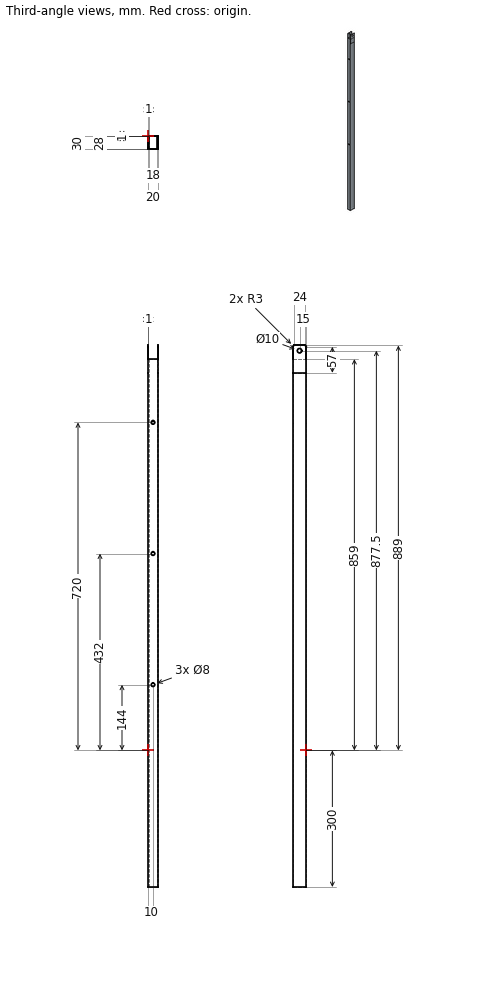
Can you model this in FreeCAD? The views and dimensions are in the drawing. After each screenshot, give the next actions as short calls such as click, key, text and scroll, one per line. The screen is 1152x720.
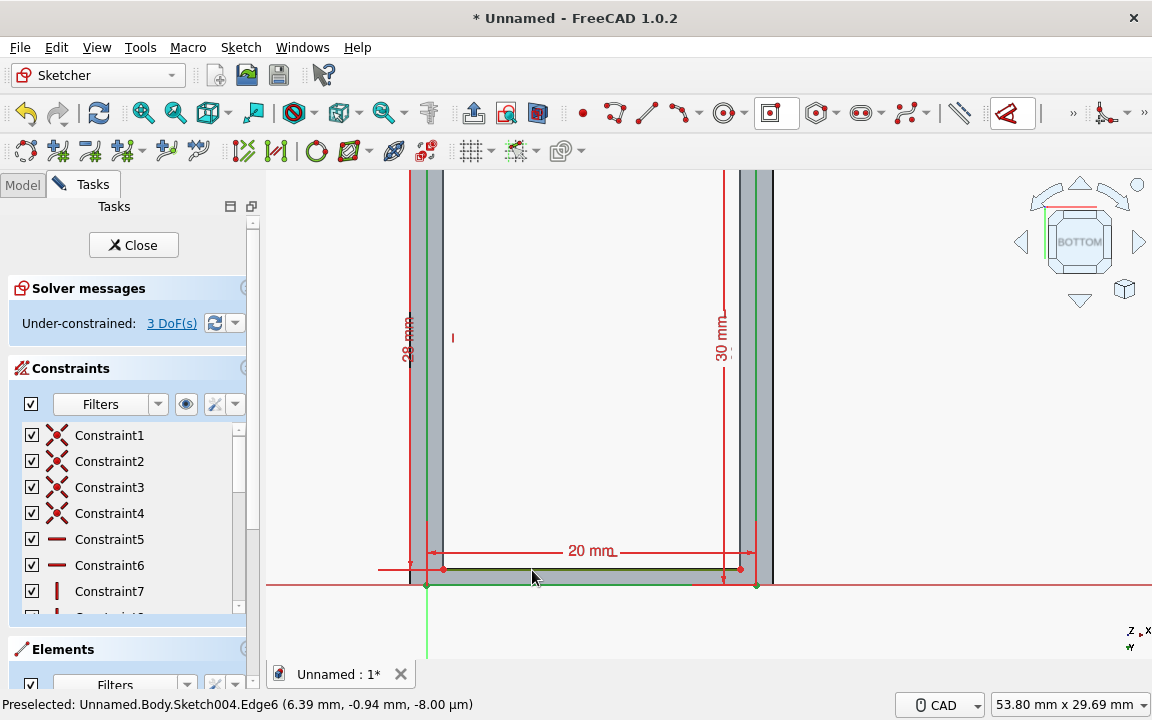
key(l)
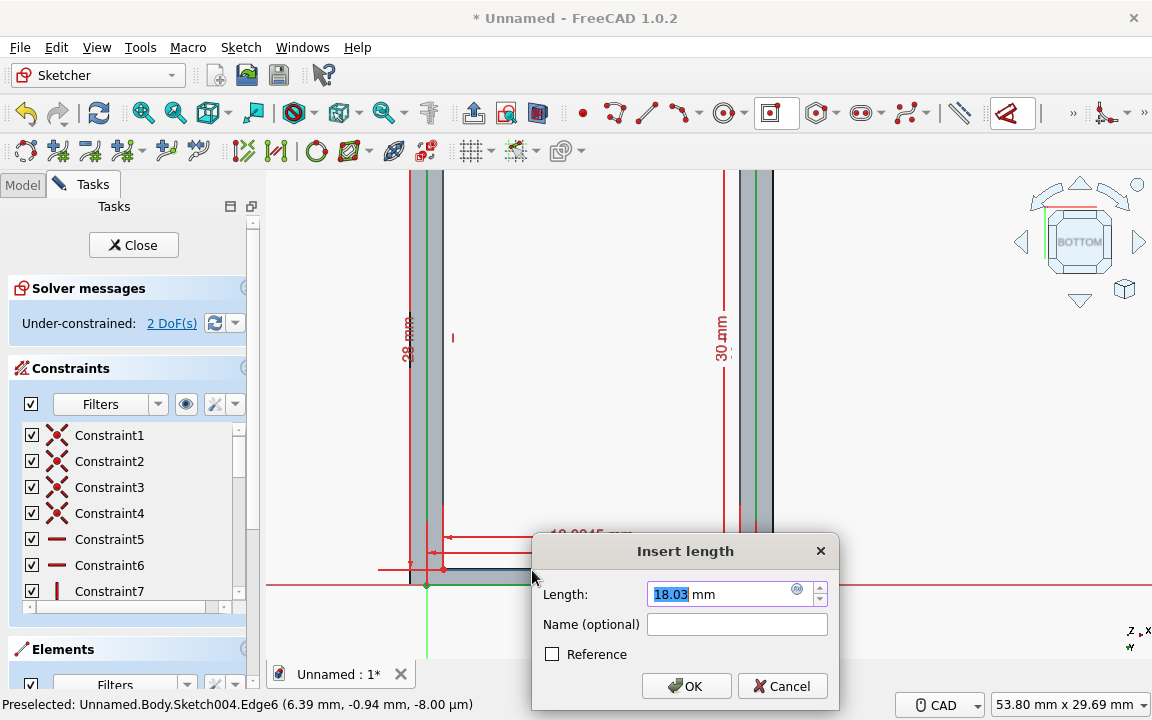
text(18)
key(Return)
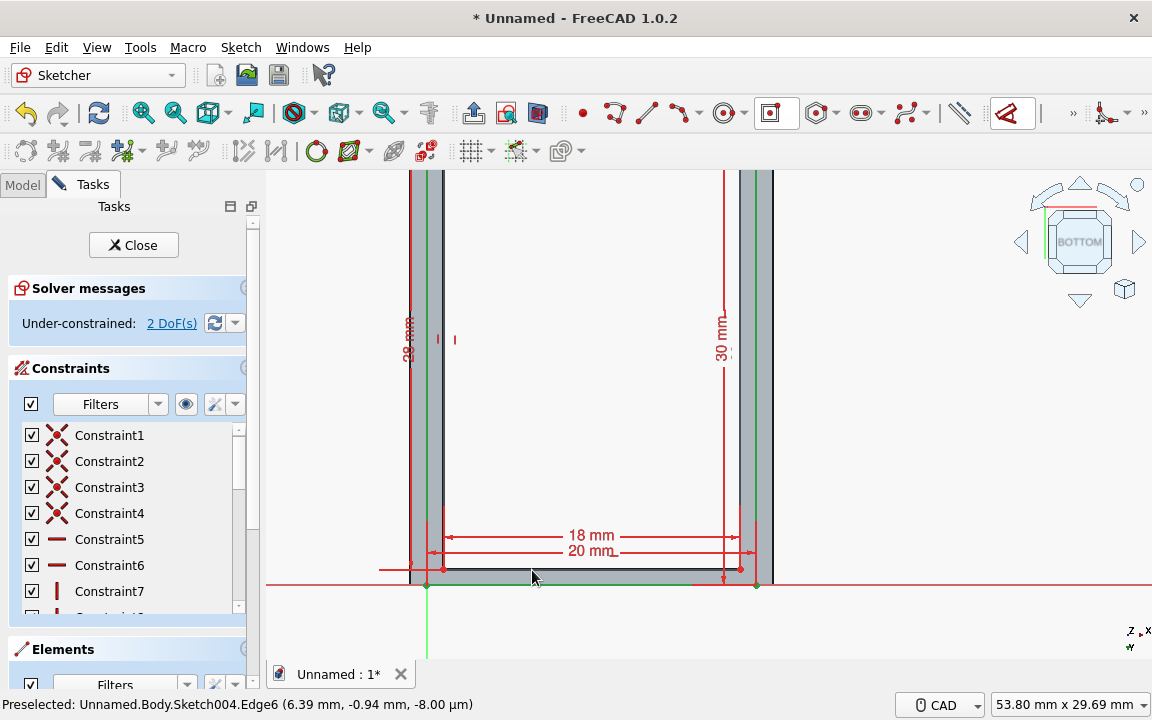
scroll(740, 569, down, 2)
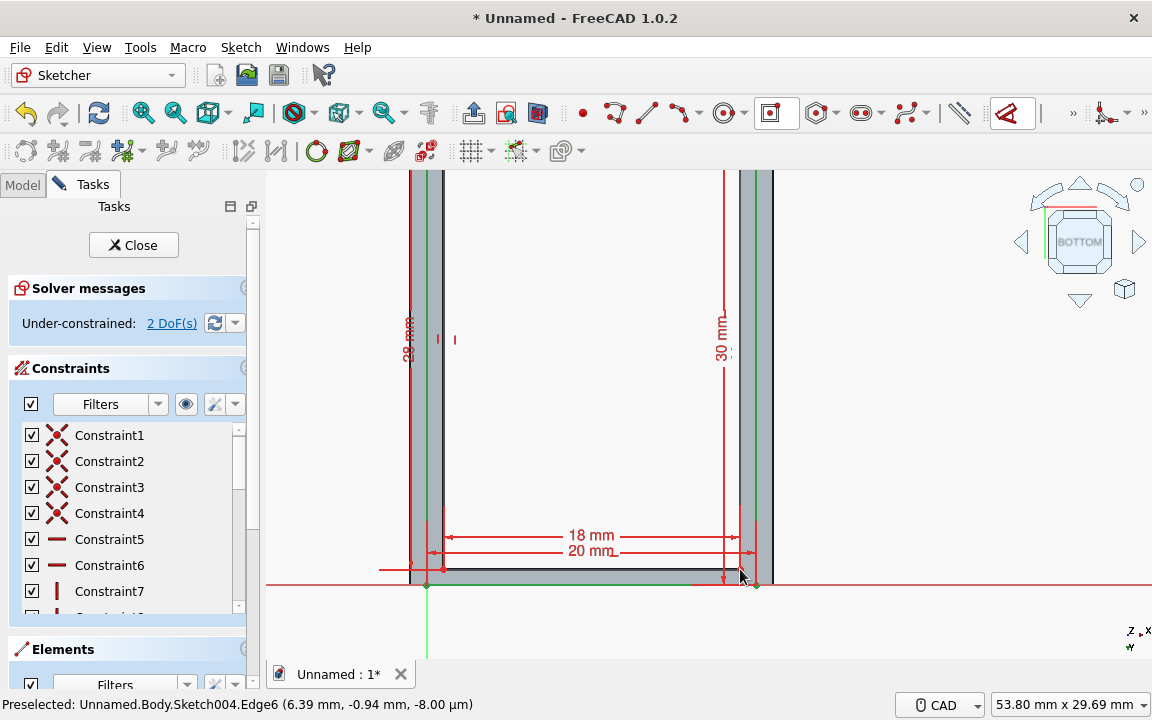
scroll(541, 261, up, 7)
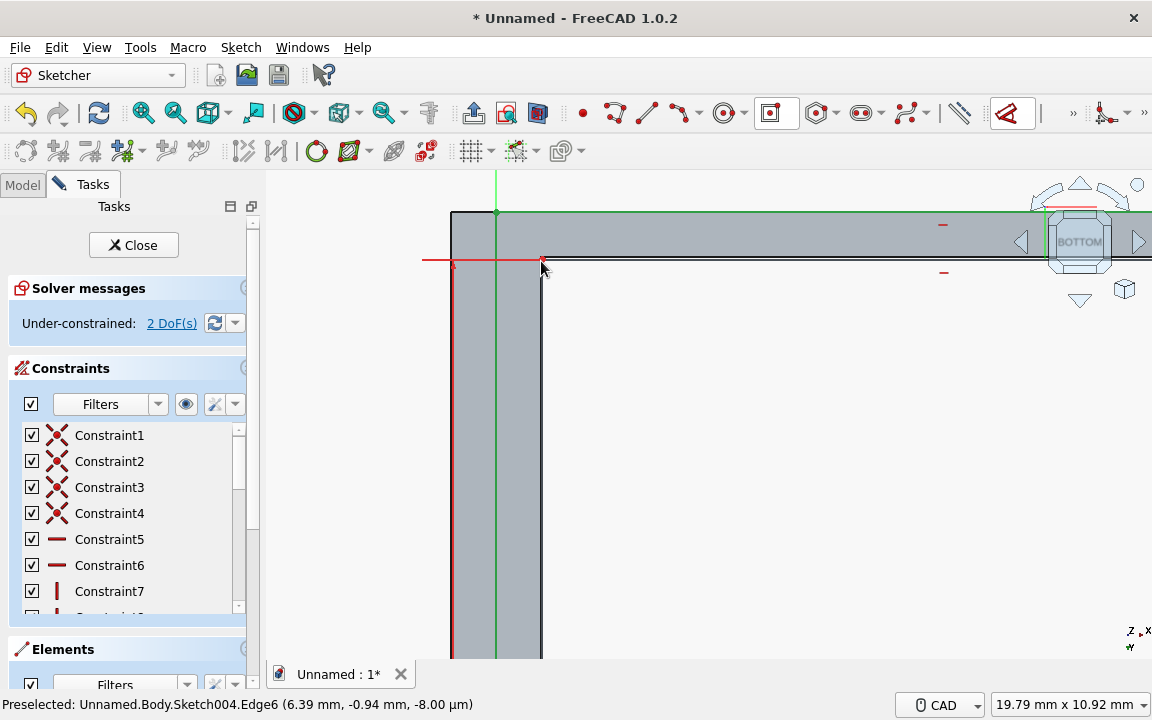
click(542, 260)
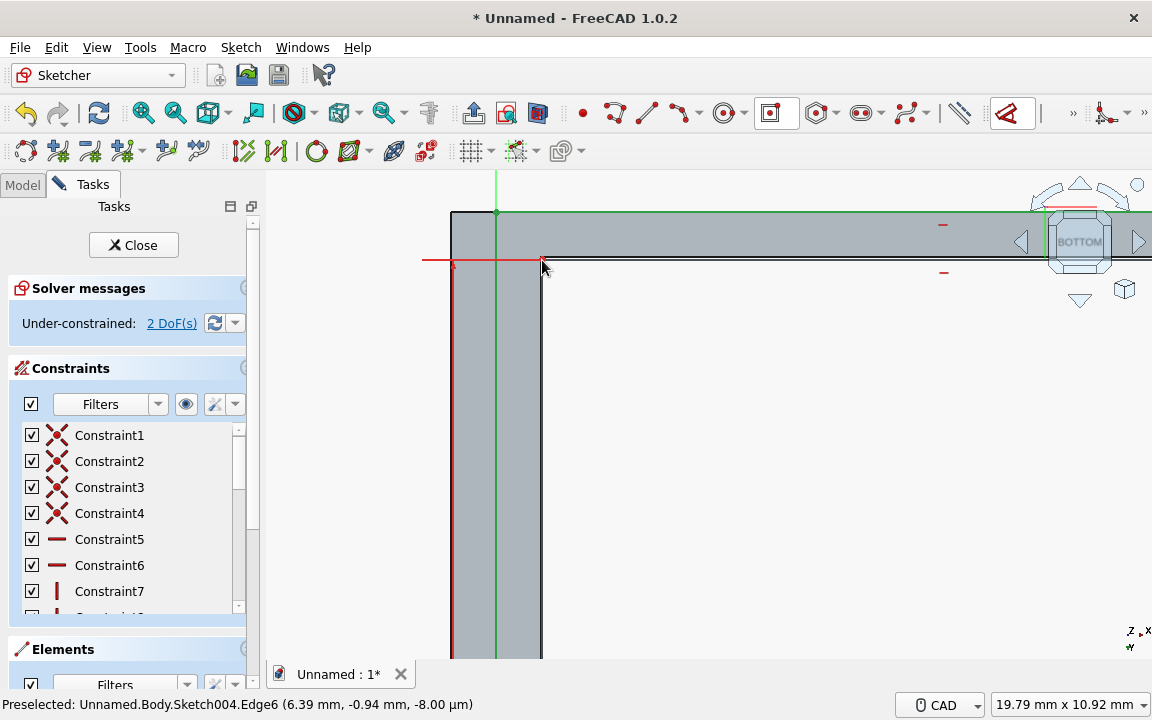
key(l)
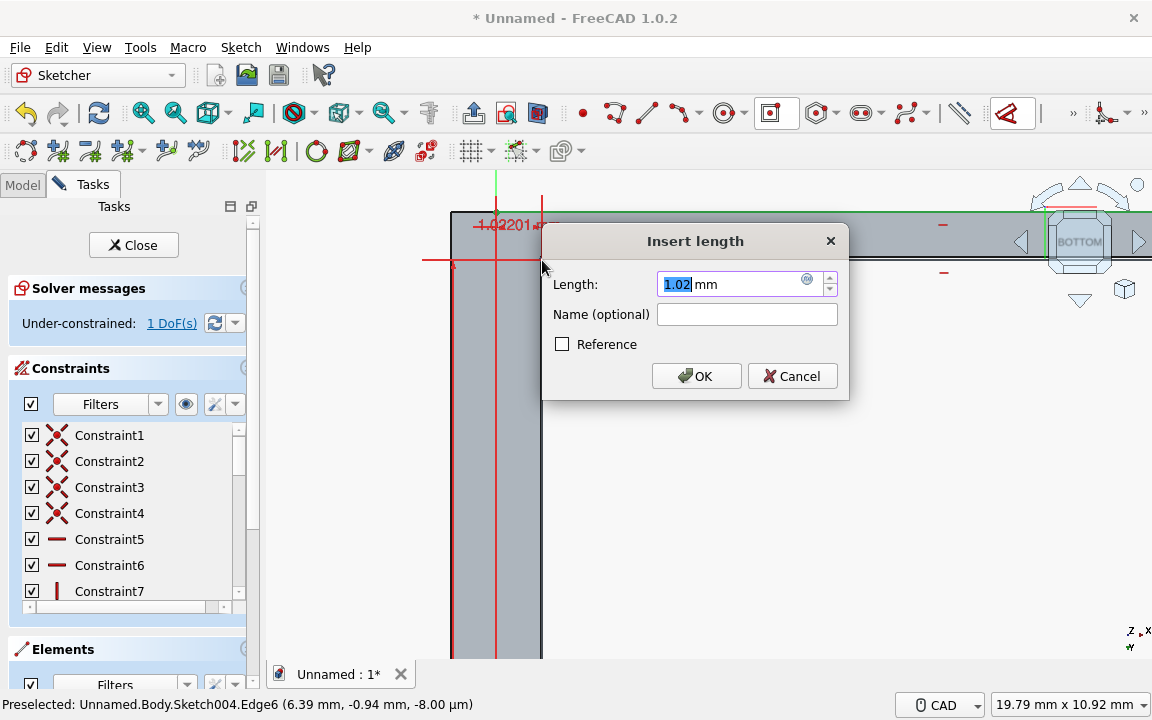
text(1)
key(Return)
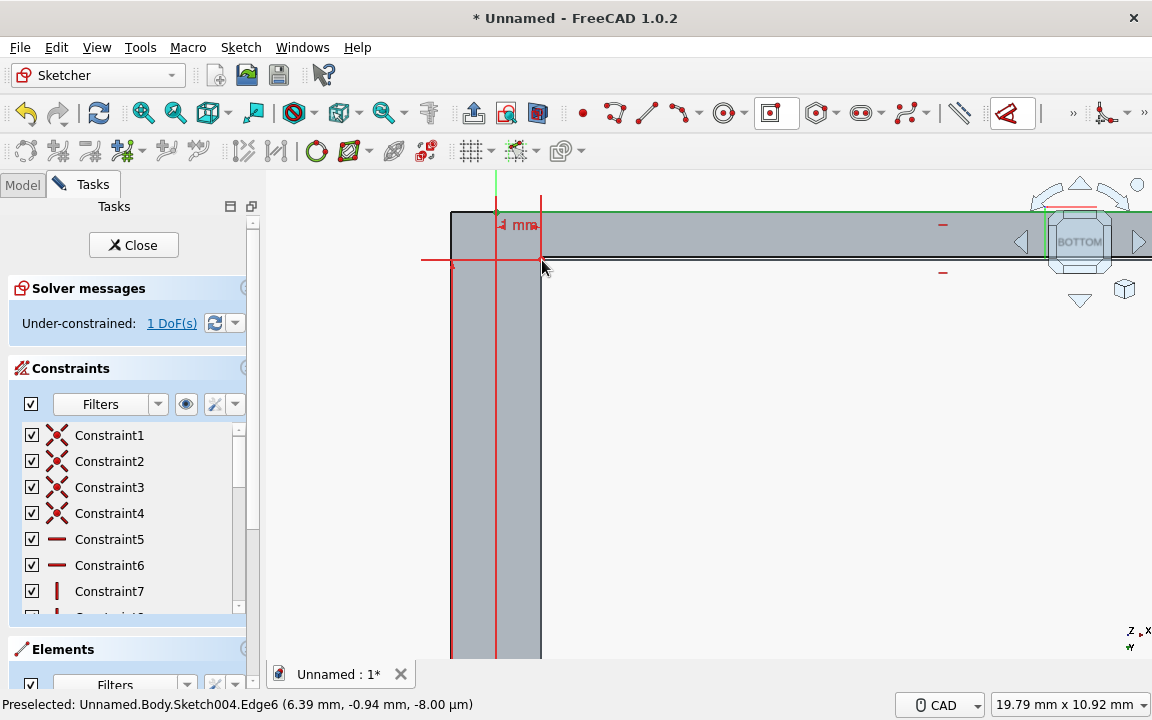
scroll(541, 261, down, 7)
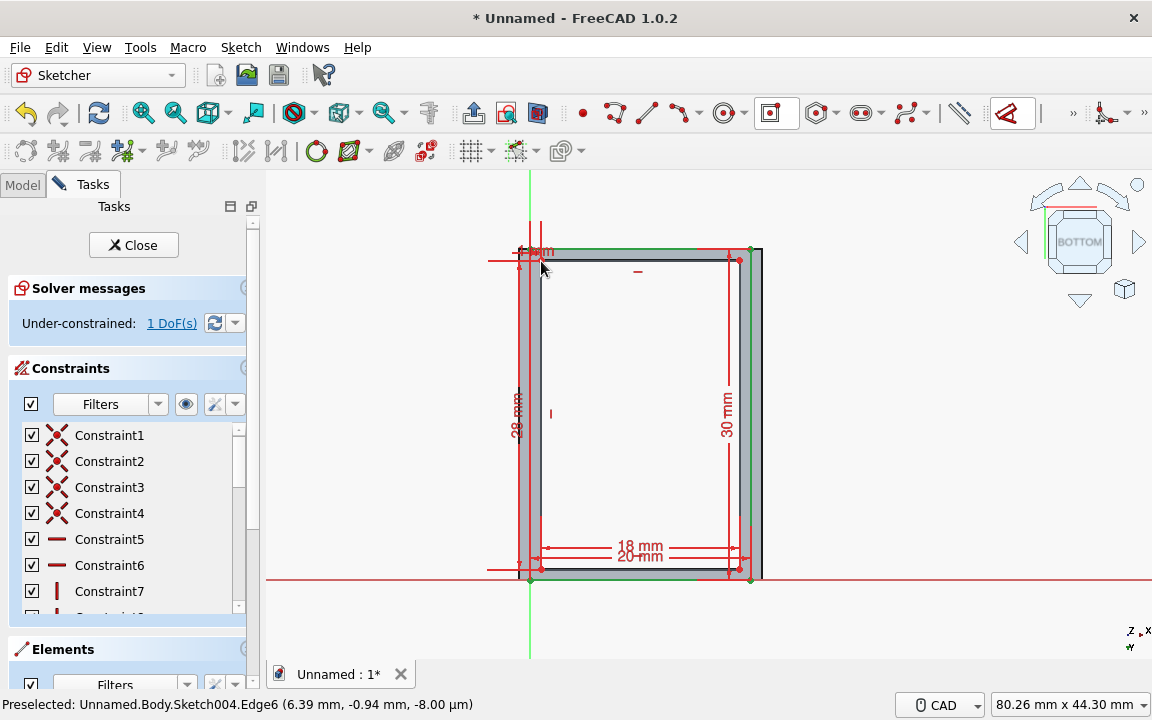
scroll(541, 570, up, 7)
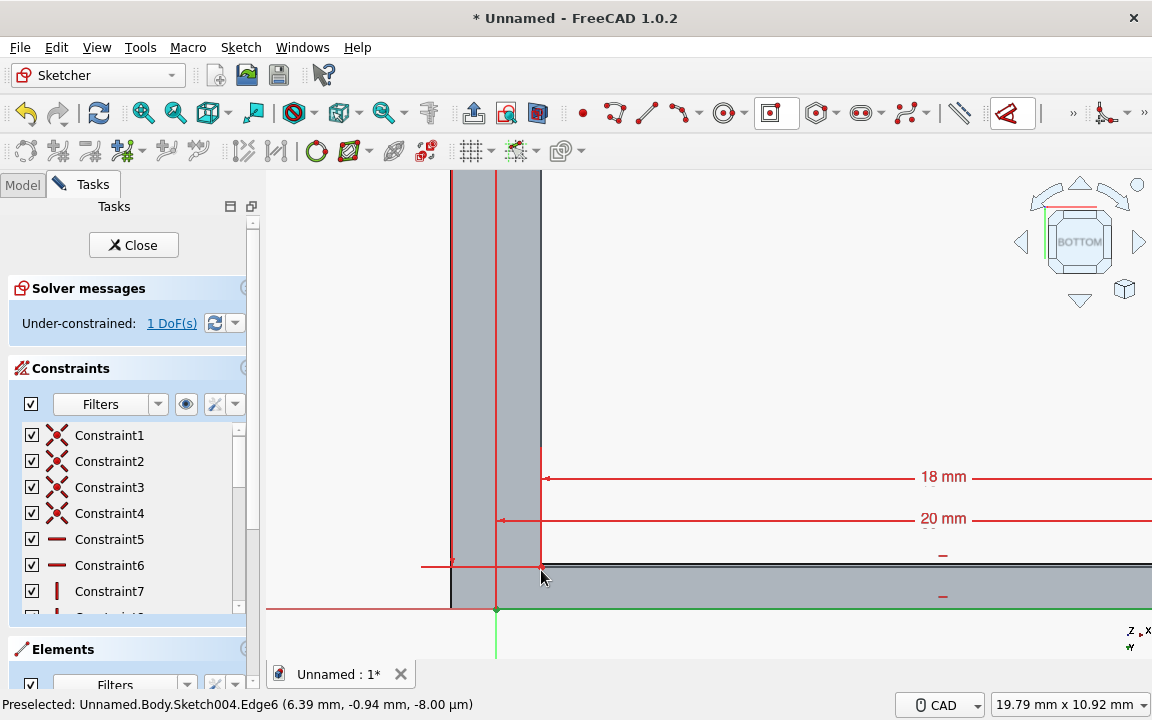
click(541, 567)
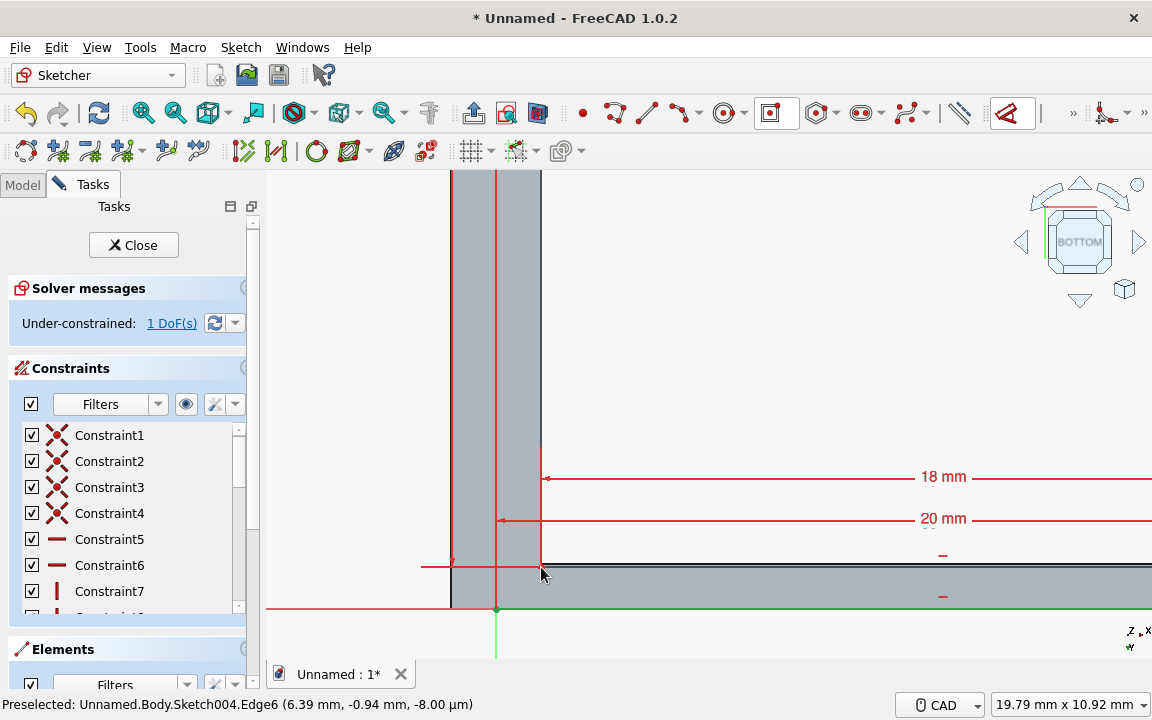
click(1030, 114)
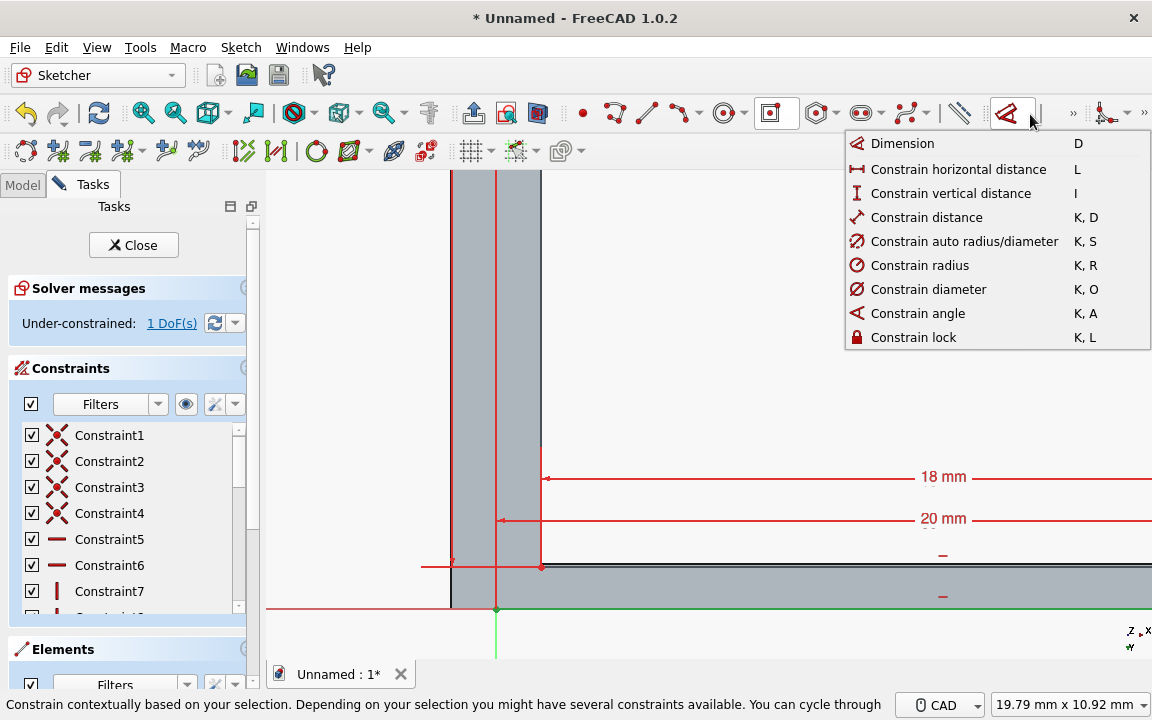
click(998, 193)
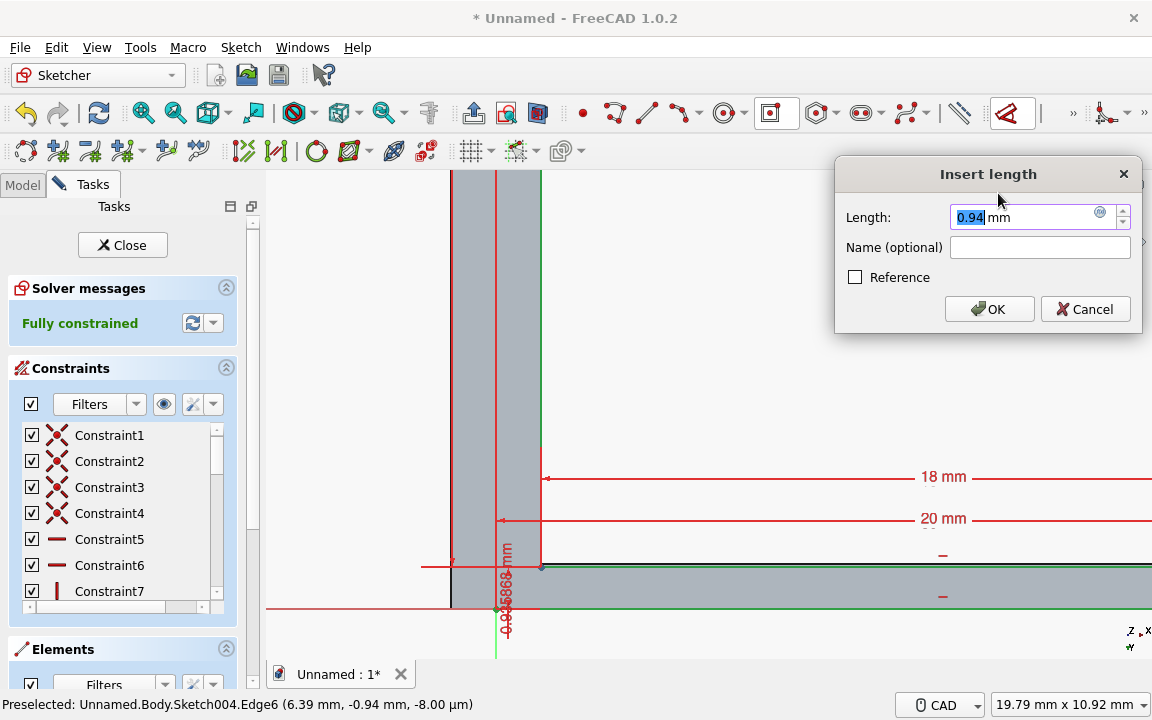
text(1)
key(Return)